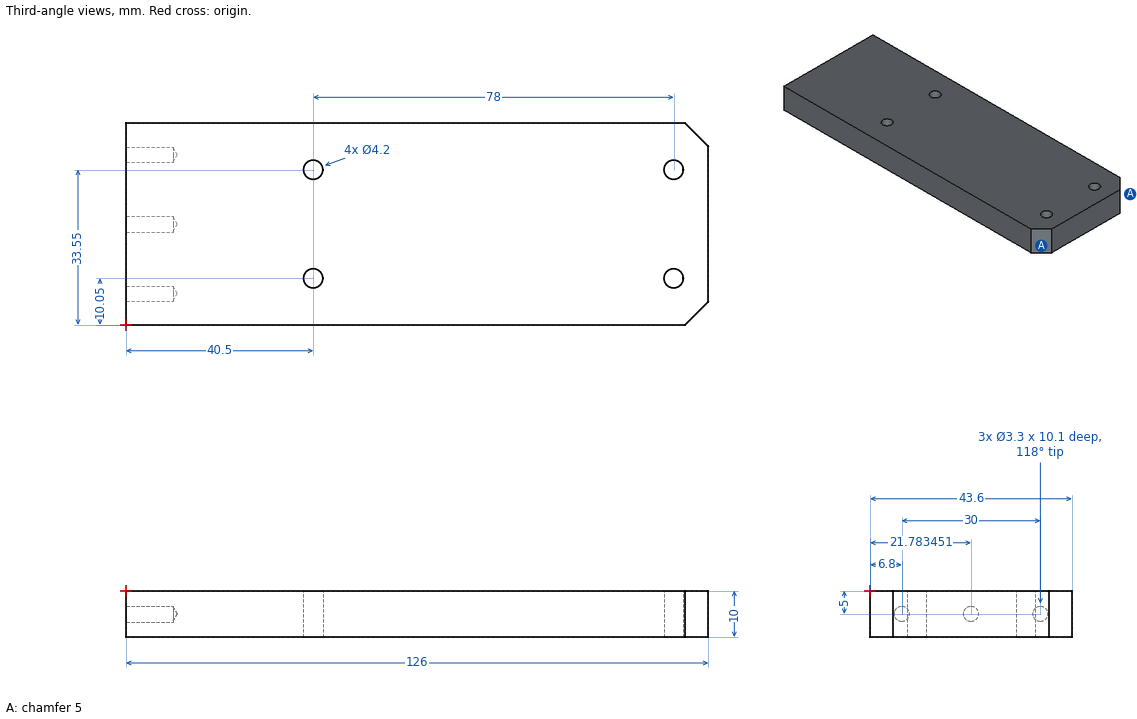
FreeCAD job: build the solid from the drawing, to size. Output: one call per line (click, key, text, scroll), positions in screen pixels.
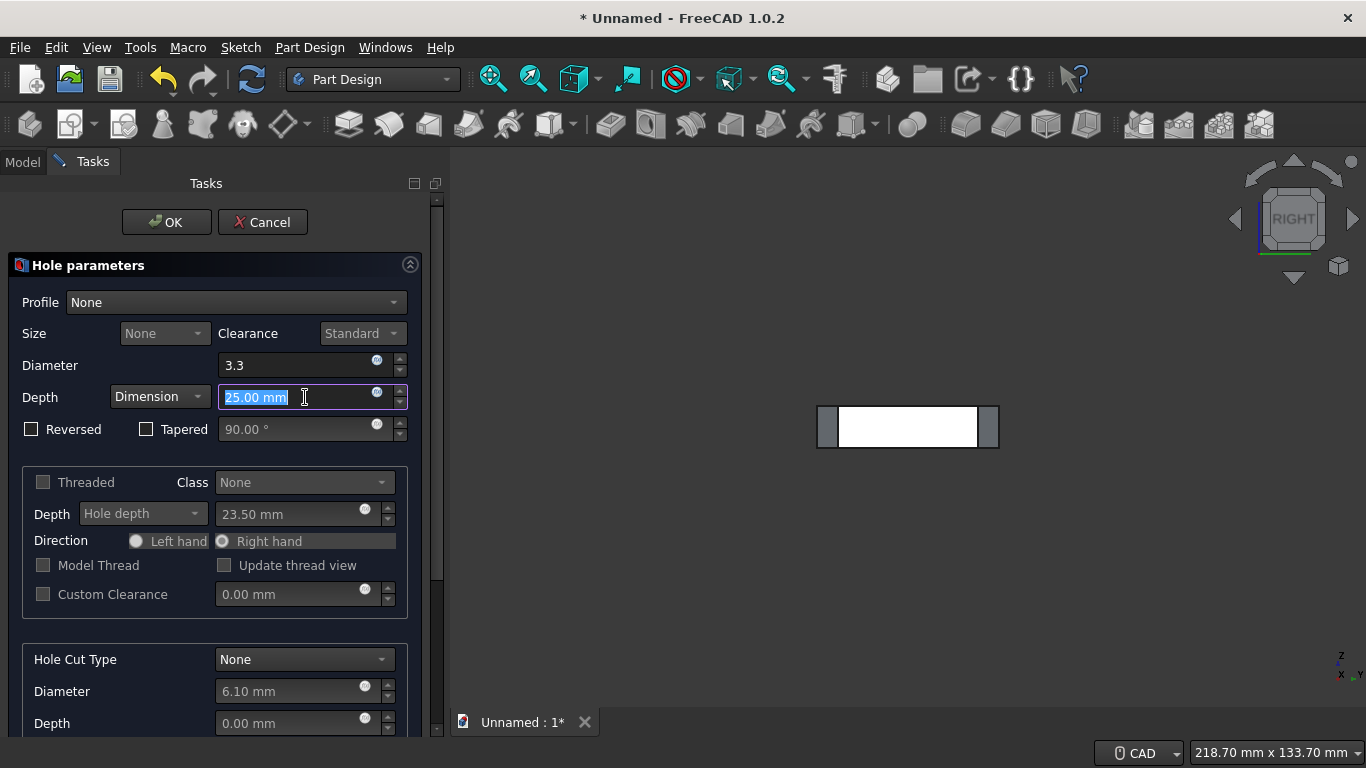
text(10.1)
key(Tab)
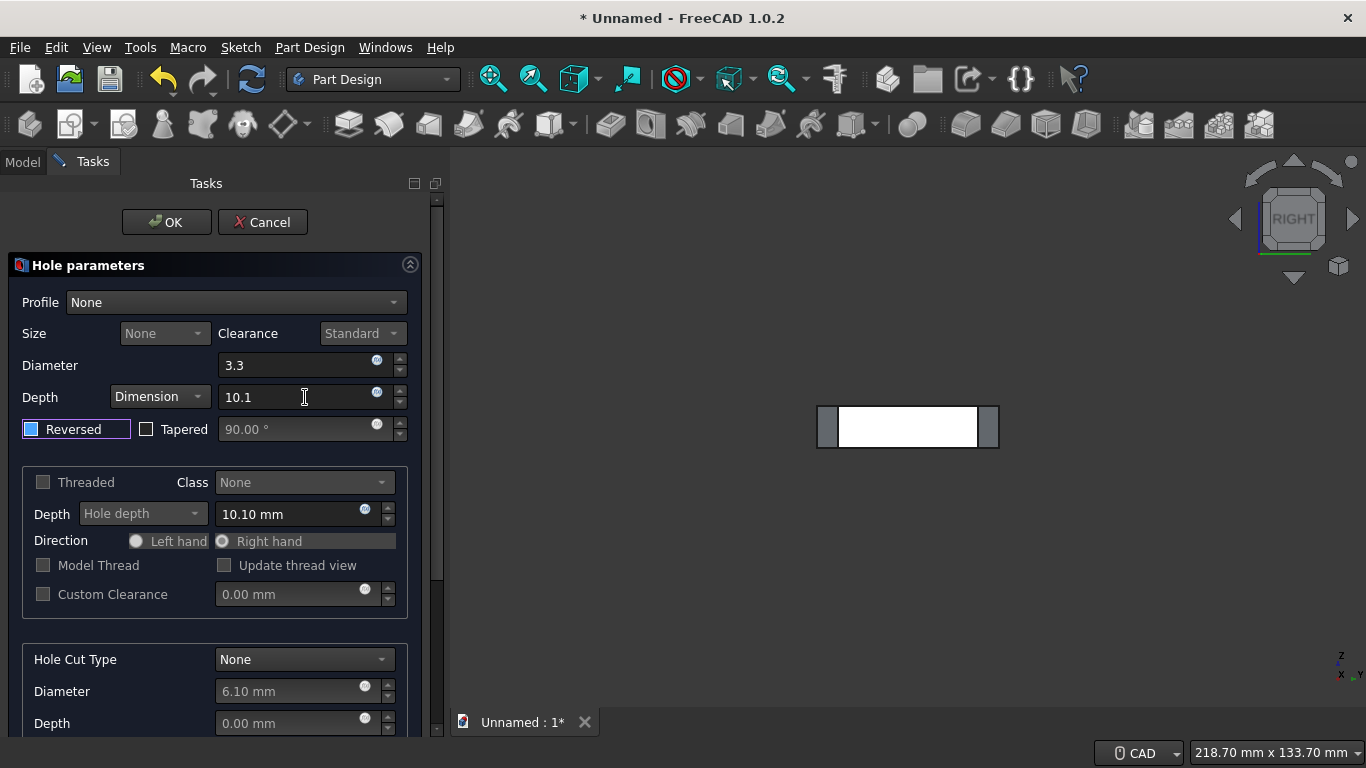
click(30, 429)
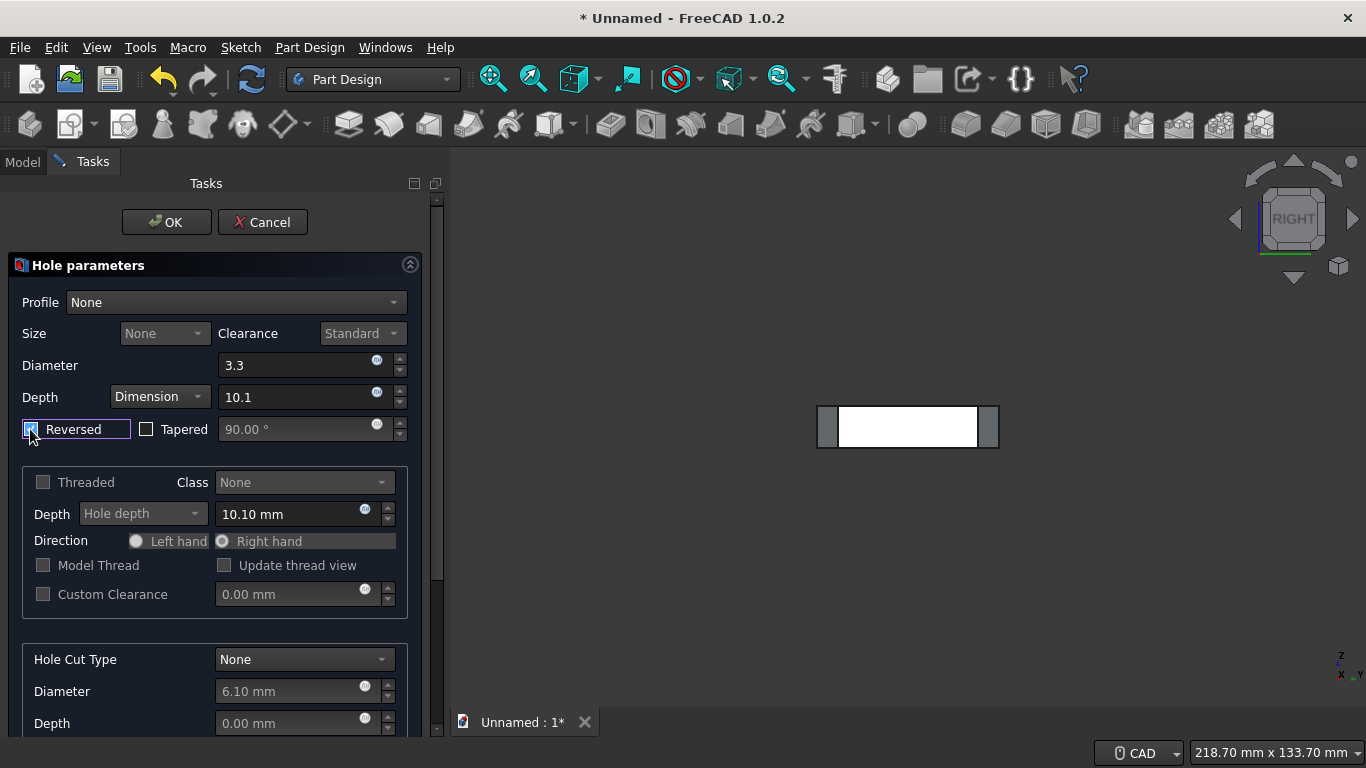
click(167, 222)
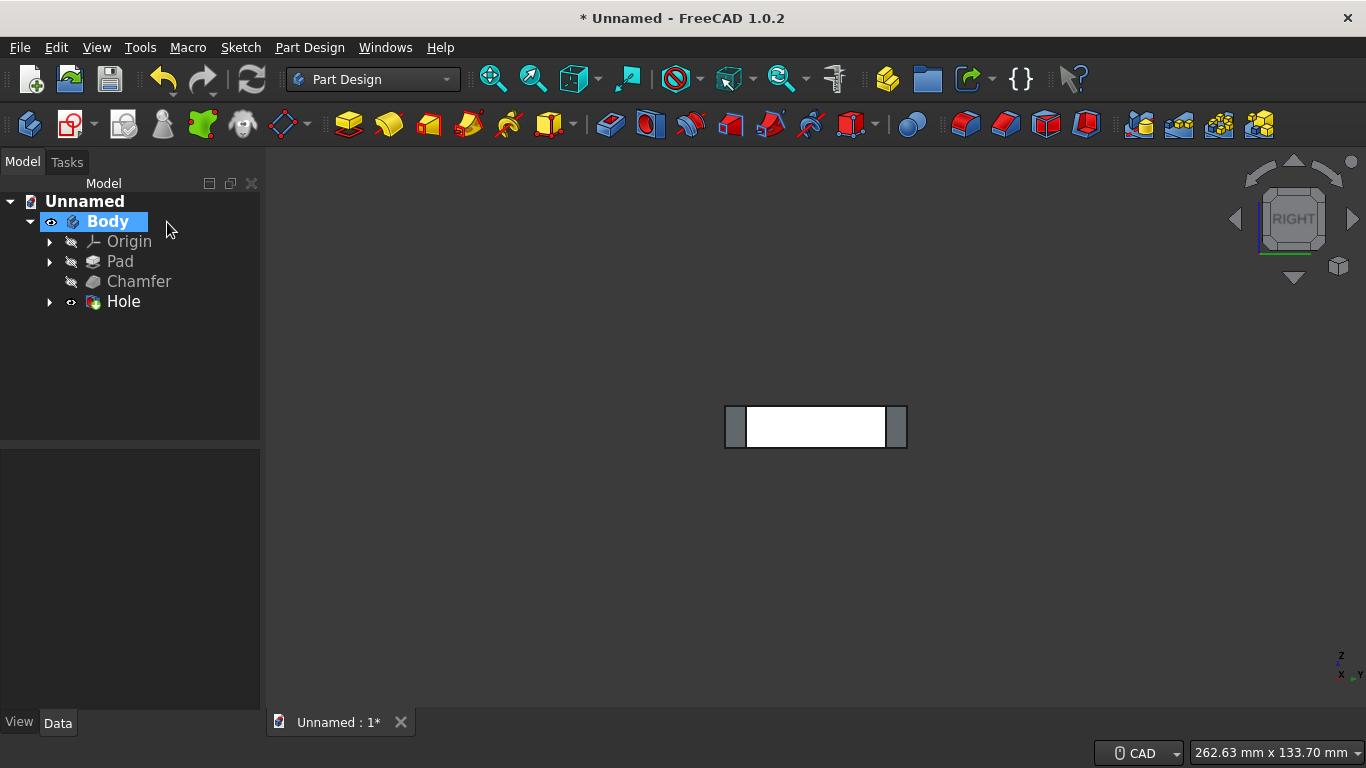
click(494, 80)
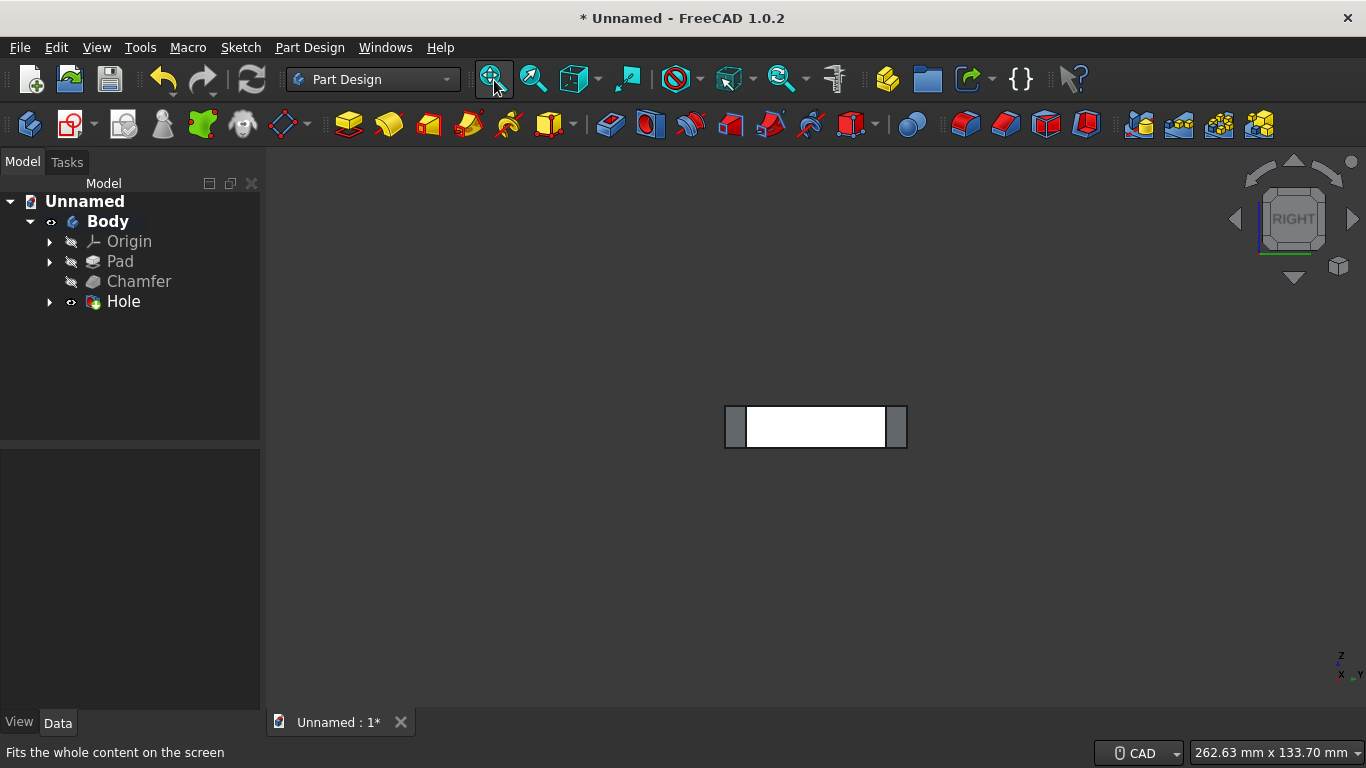
key(5)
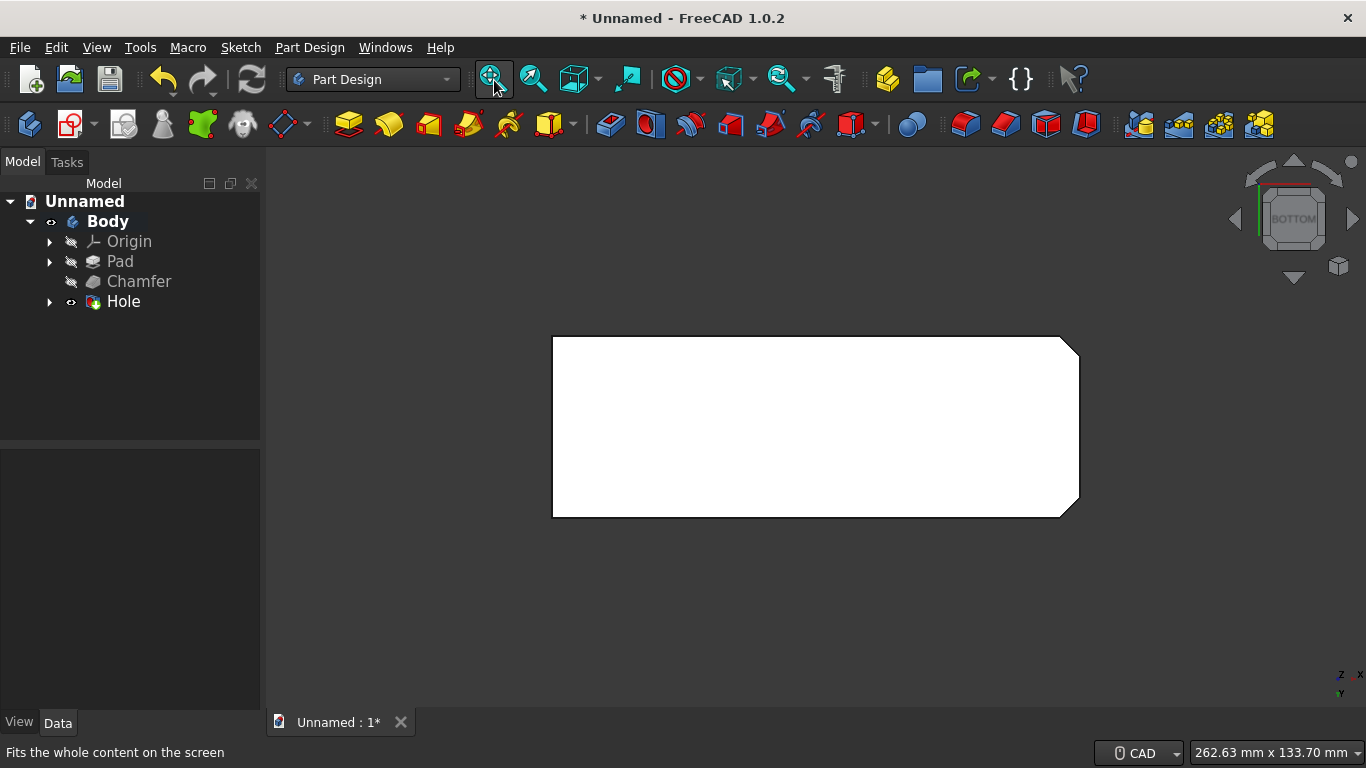
click(967, 426)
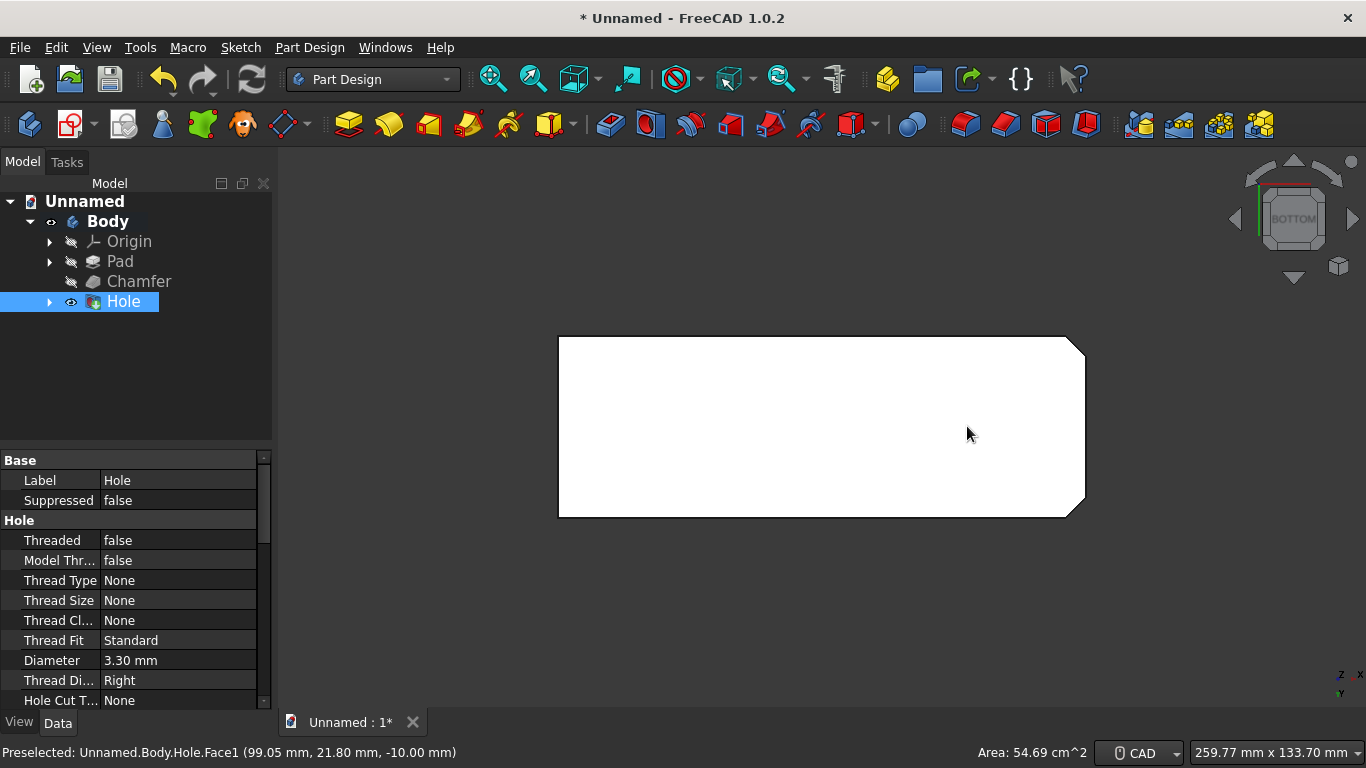
click(70, 124)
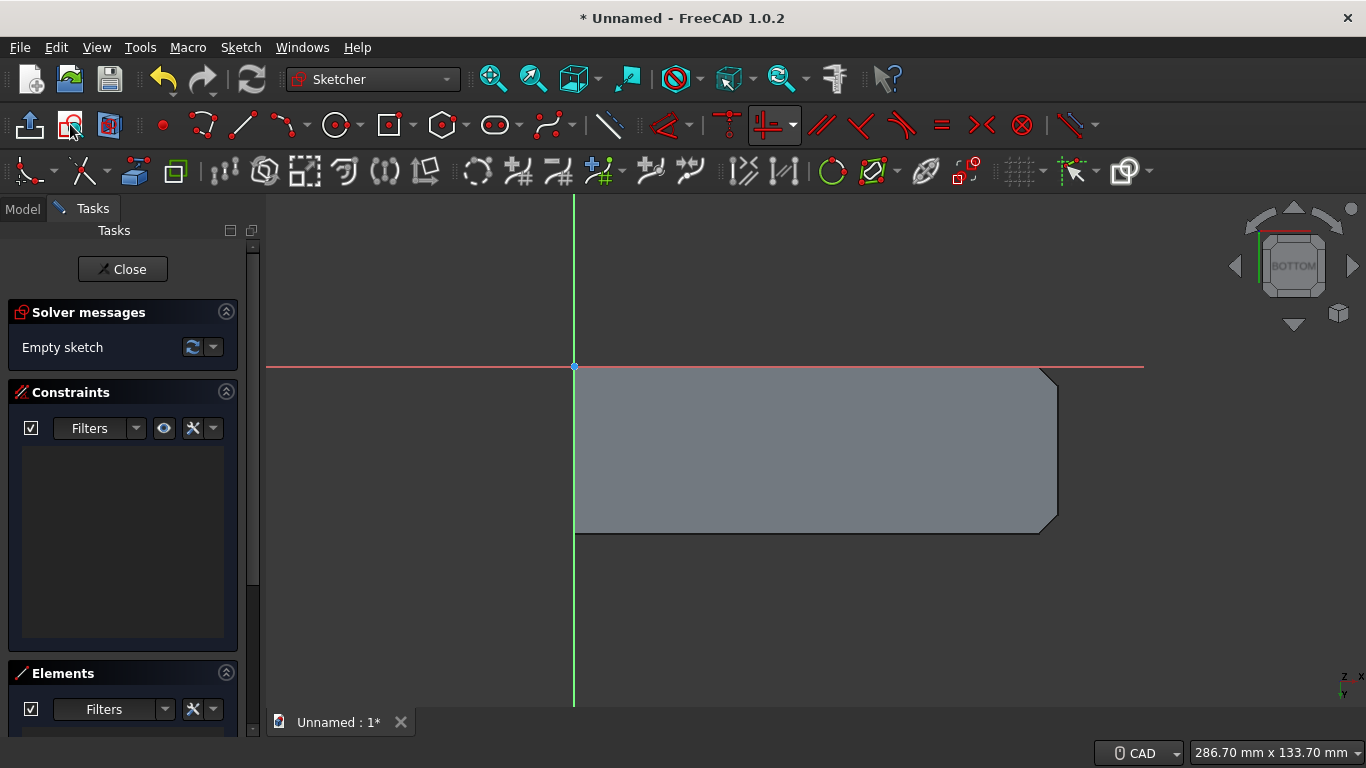
scroll(924, 404, up, 2)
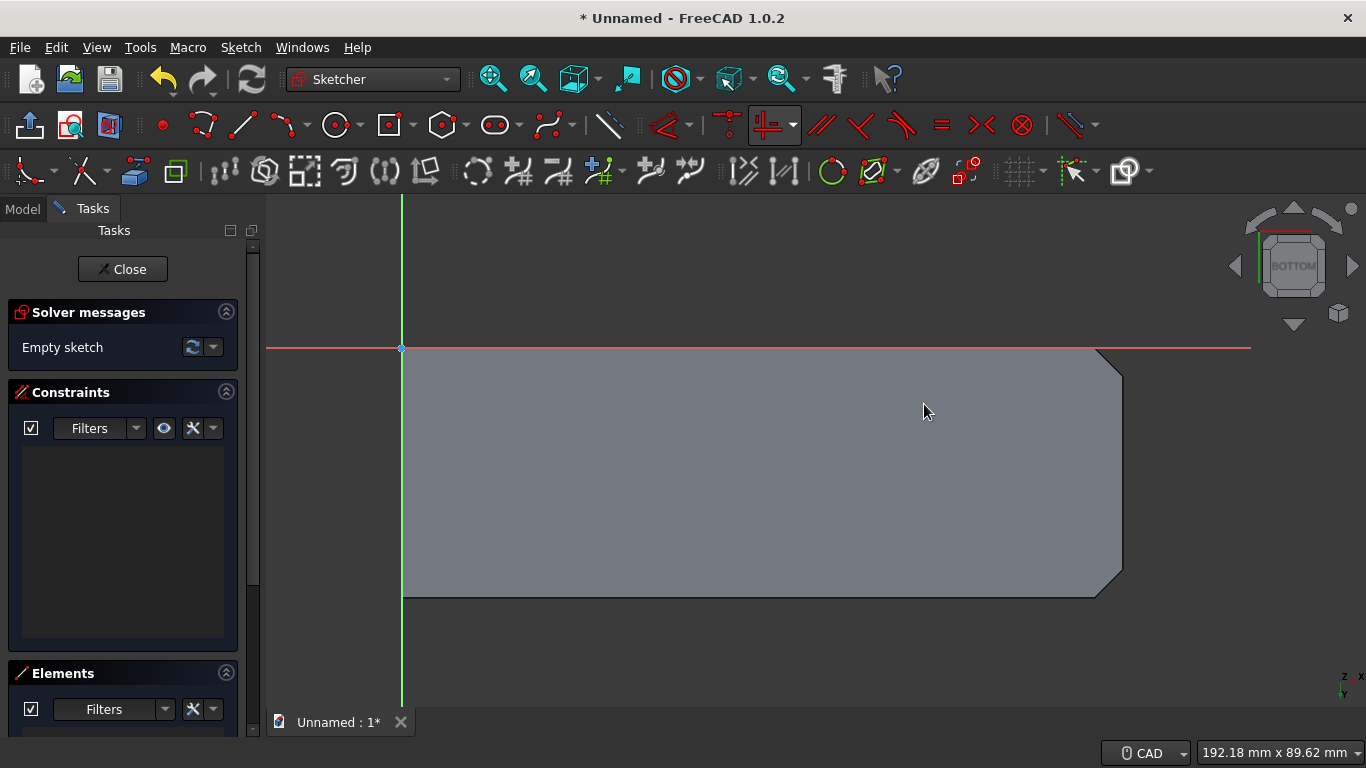
click(336, 126)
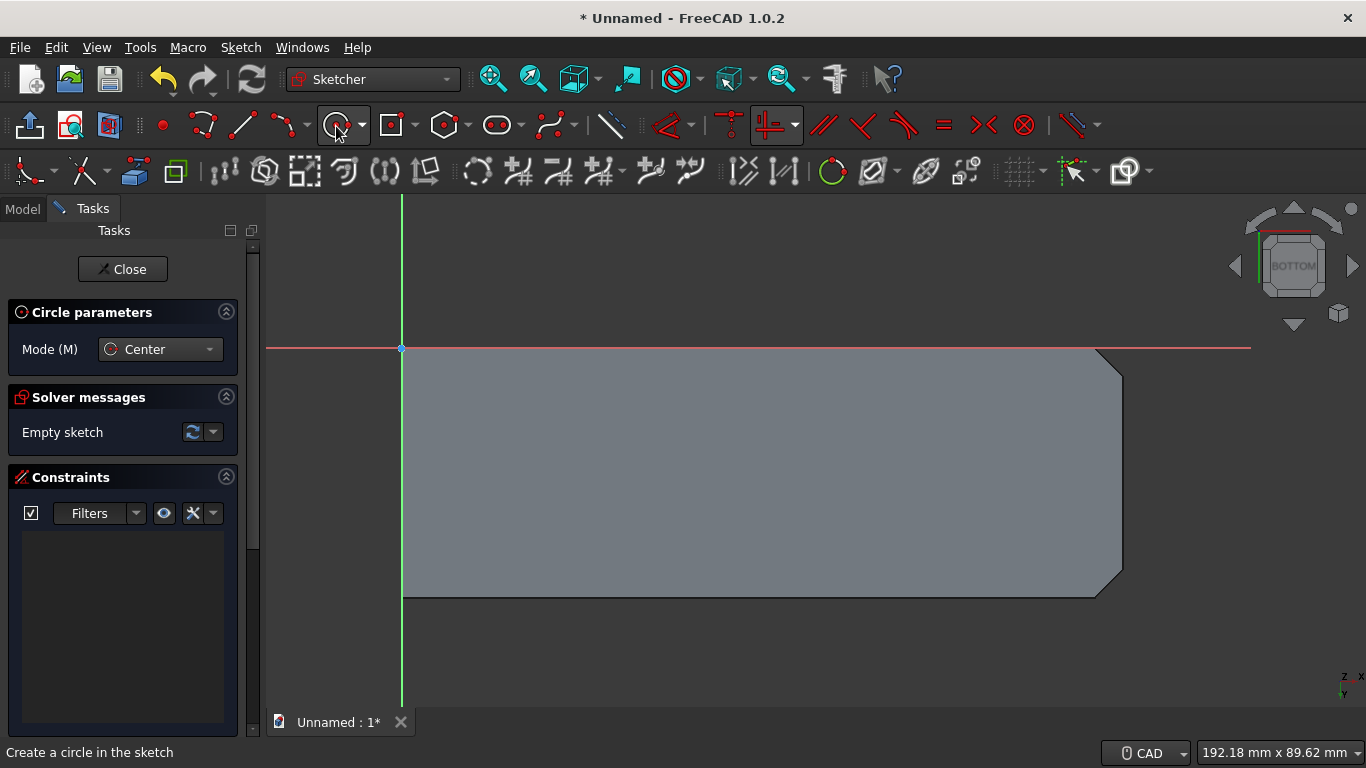
scroll(634, 540, up, 4)